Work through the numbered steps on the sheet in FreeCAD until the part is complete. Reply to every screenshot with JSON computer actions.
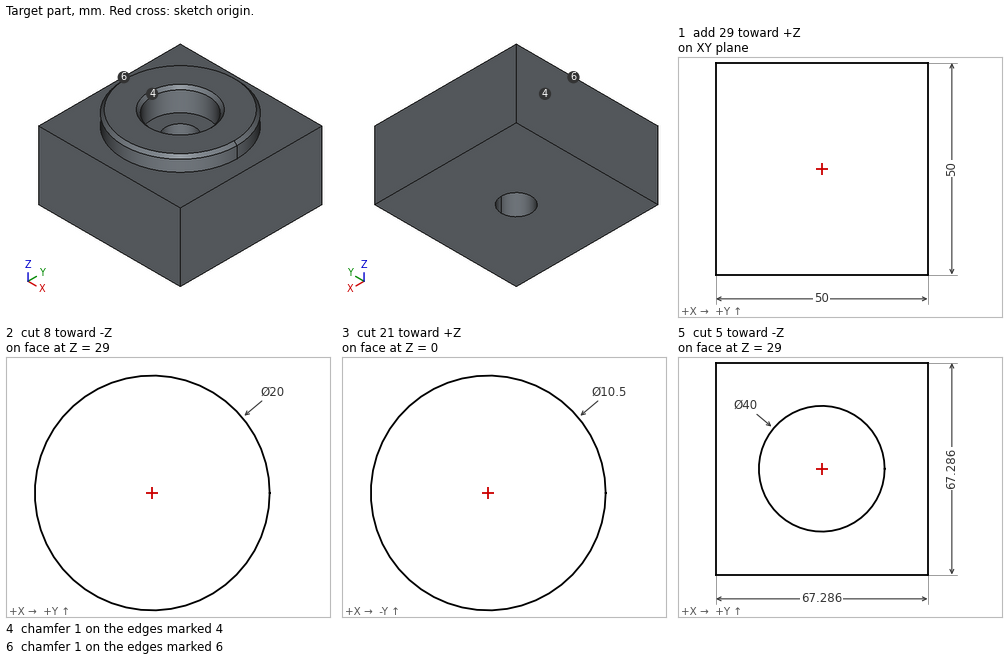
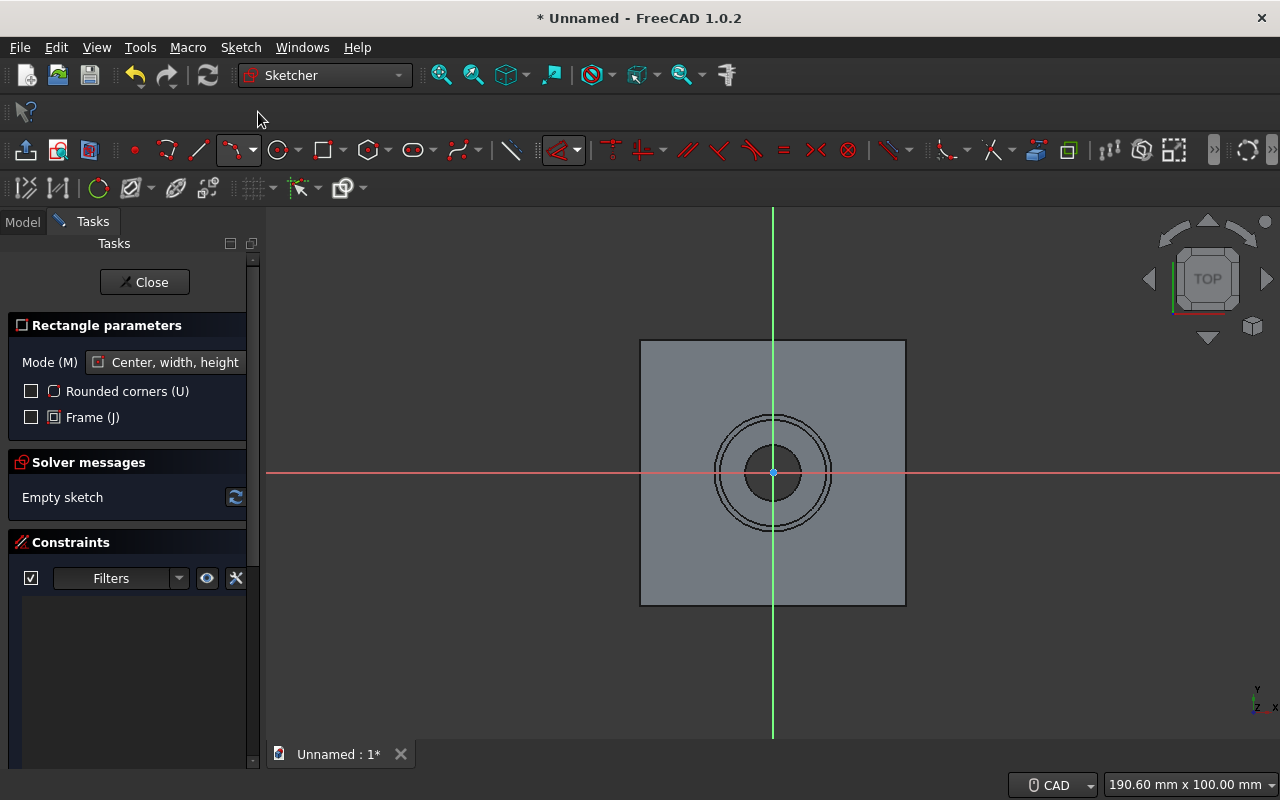
{"action": "left_click", "coordinate": [773, 473]}
{"action": "mouse_move", "coordinate": [952, 294]}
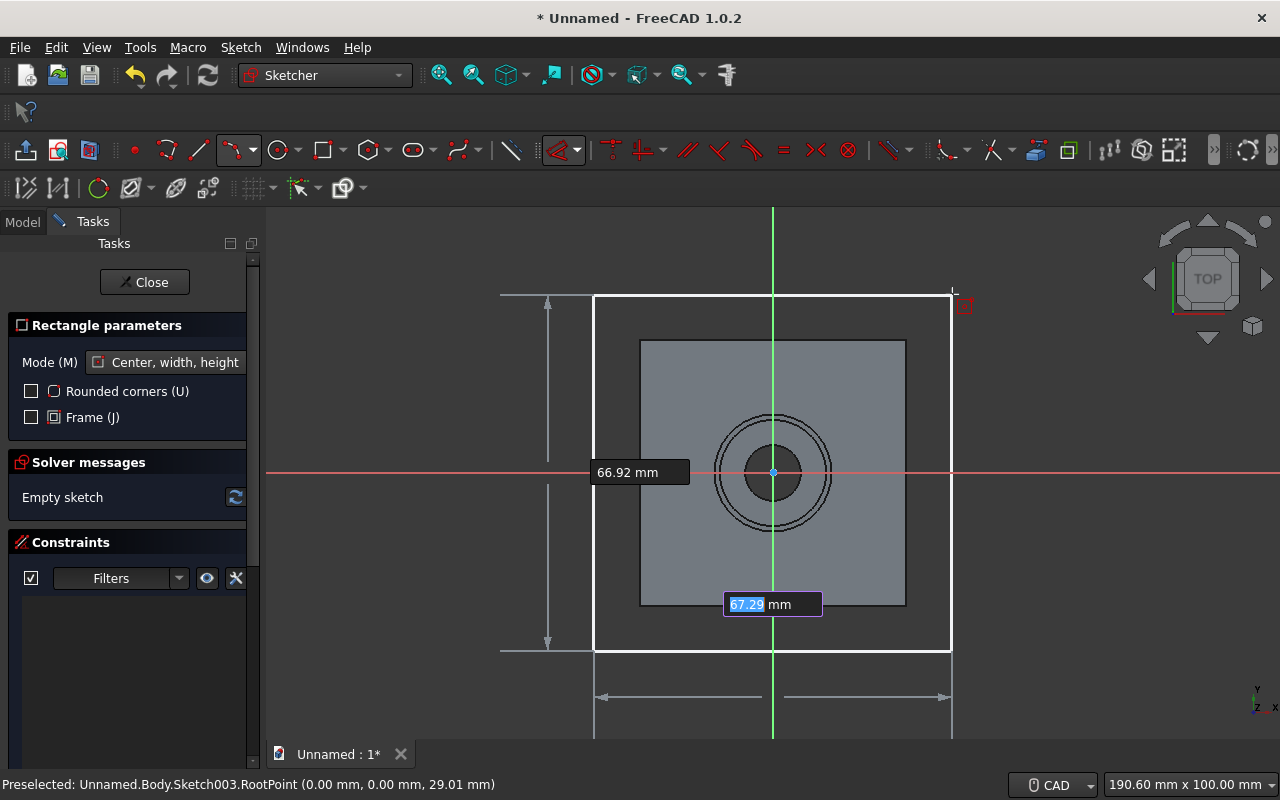
{"action": "type", "text": "67.286"}
{"action": "key", "text": "Tab"}
{"action": "type", "text": "67.286"}
{"action": "key", "text": "Return"}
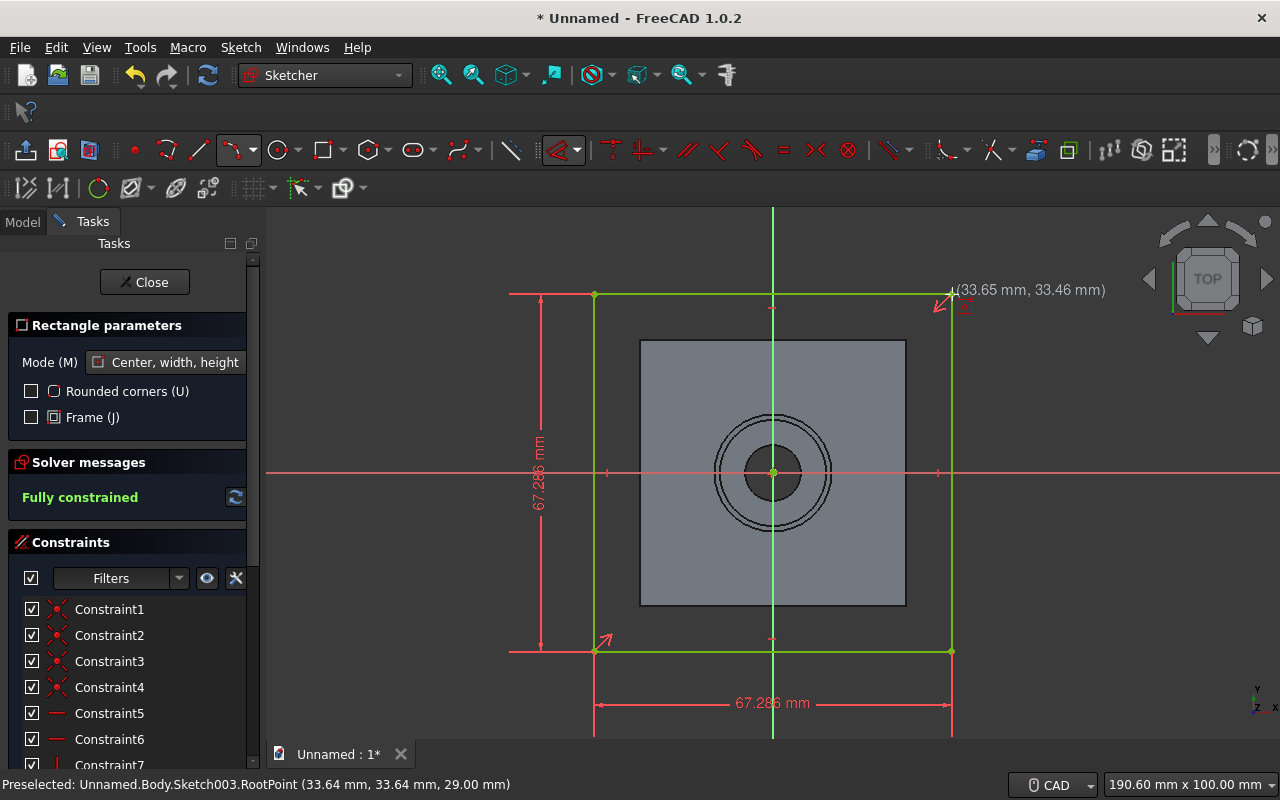
{"action": "left_click", "coordinate": [278, 150]}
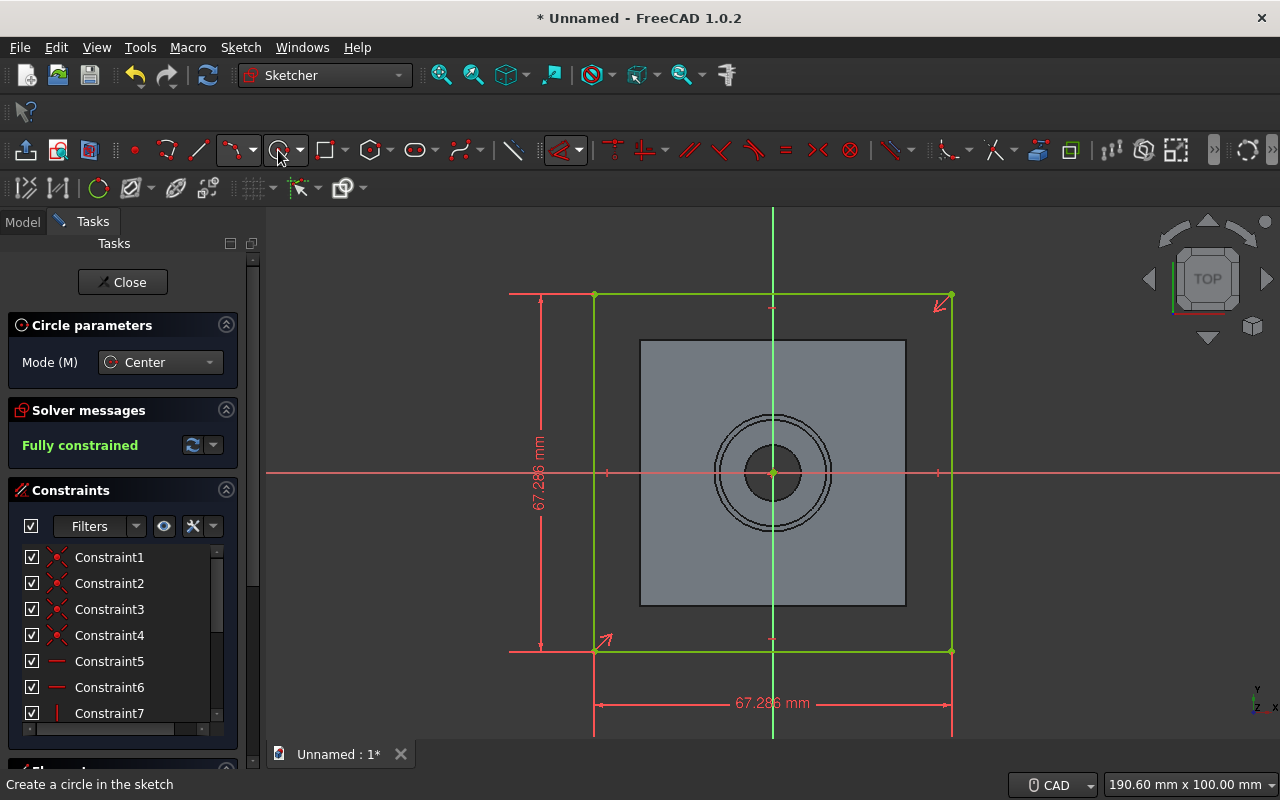
{"action": "left_click", "coordinate": [773, 473]}
{"action": "mouse_move", "coordinate": [848, 398]}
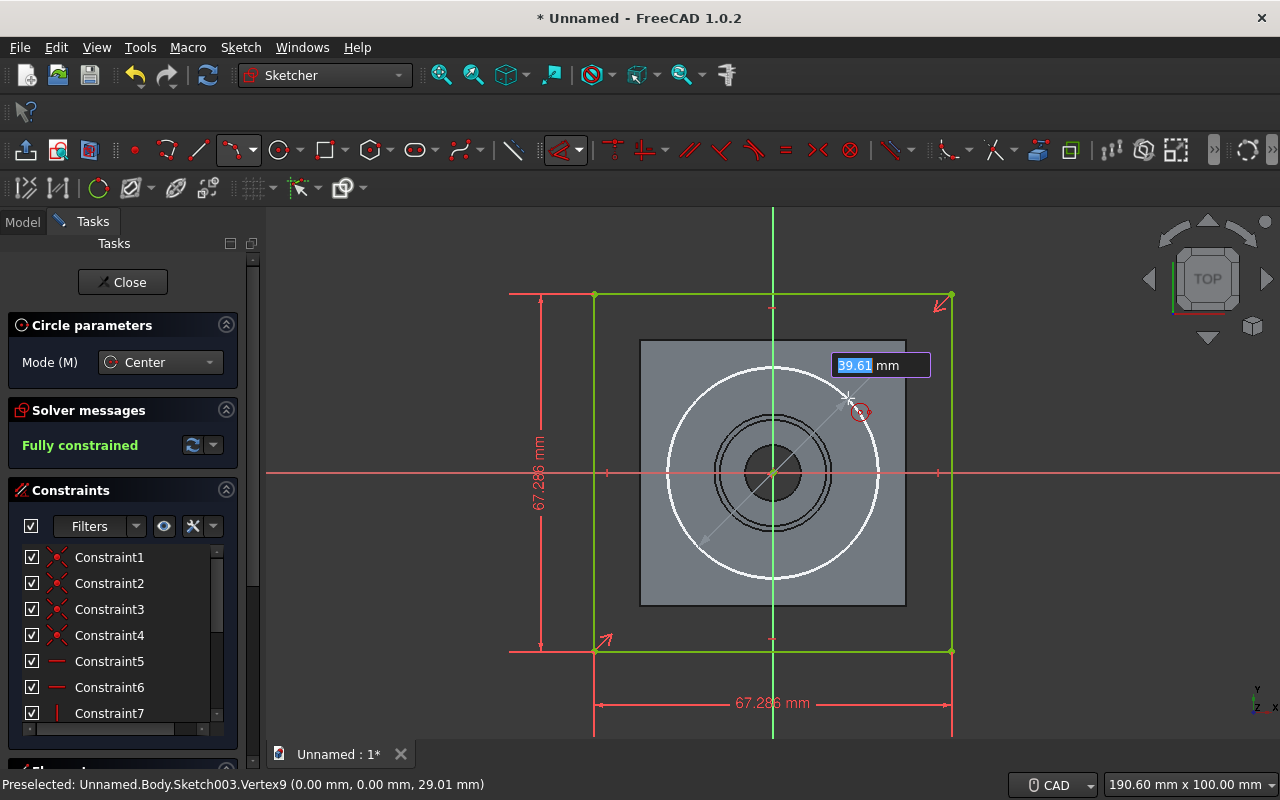
{"action": "type", "text": "40"}
{"action": "key", "text": "Return"}
{"action": "key", "text": "Escape"}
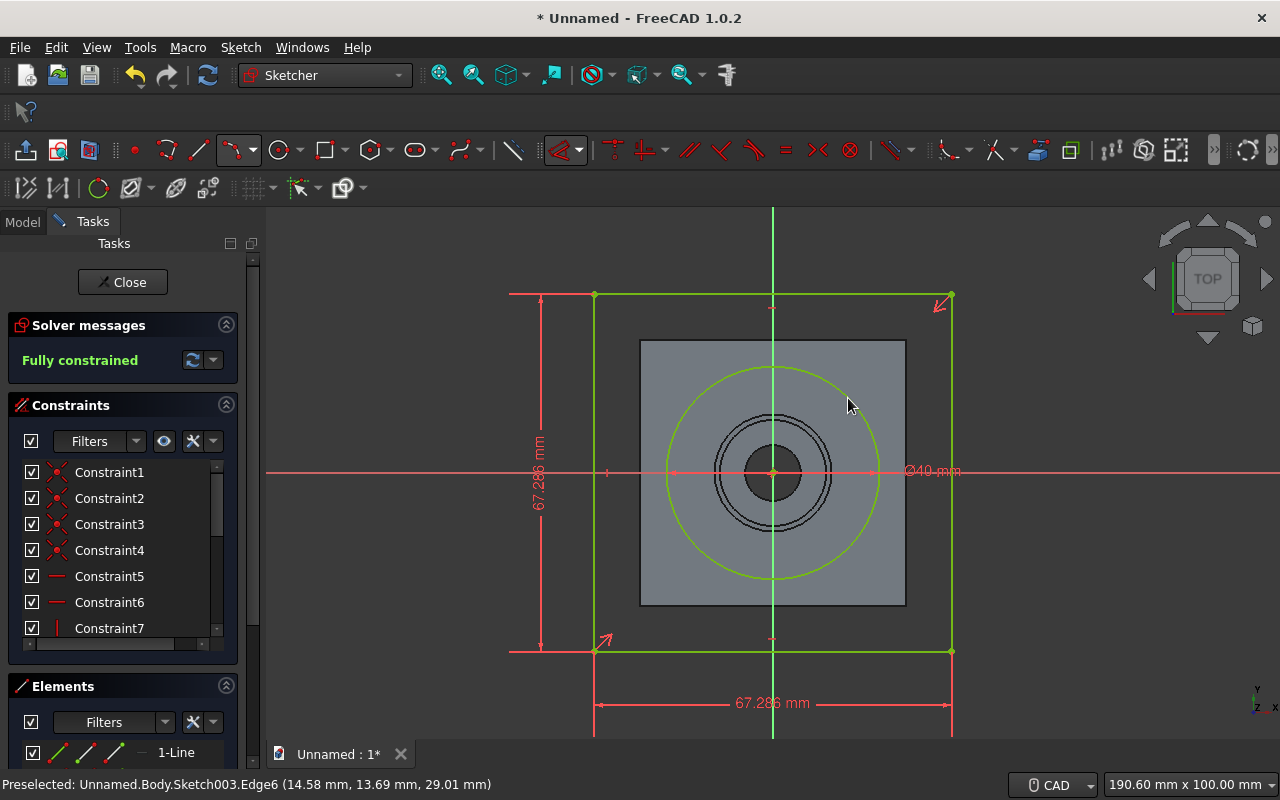
{"action": "left_click", "coordinate": [123, 282]}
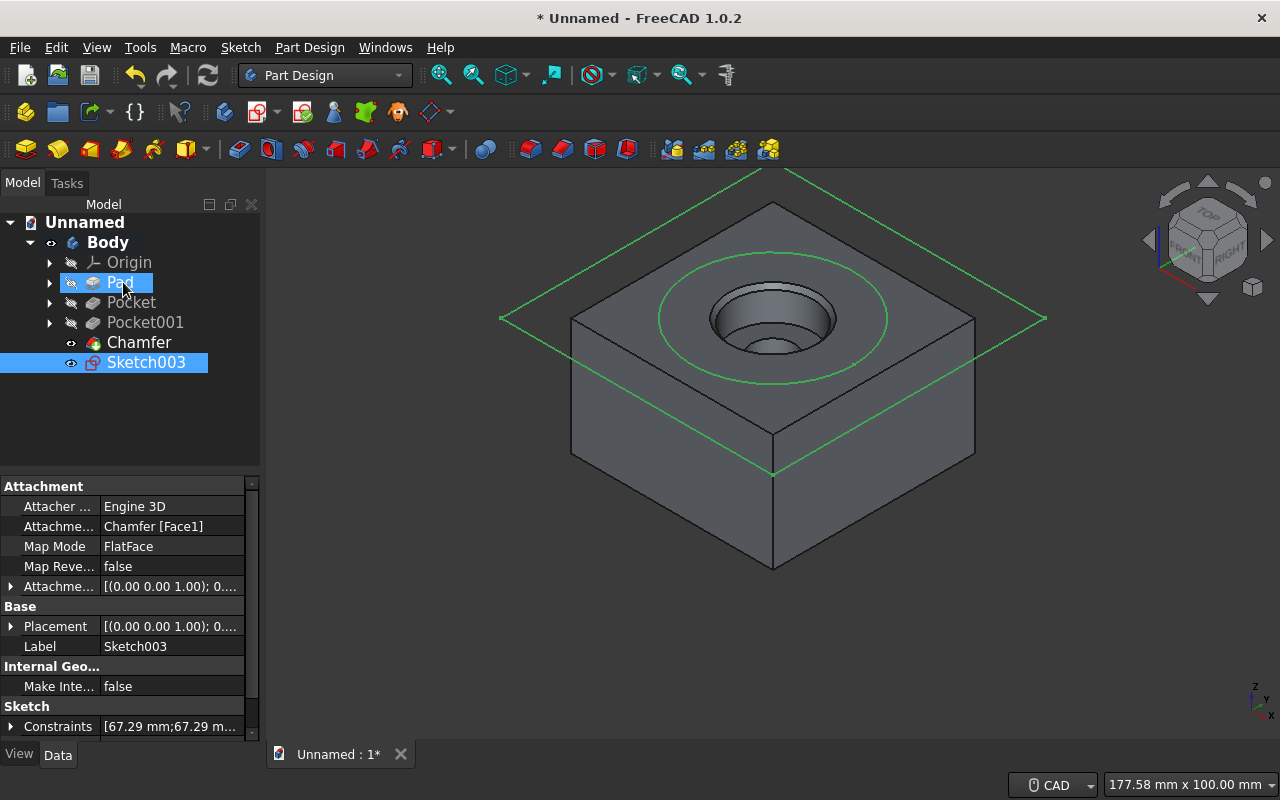
{"action": "left_click", "coordinate": [240, 150]}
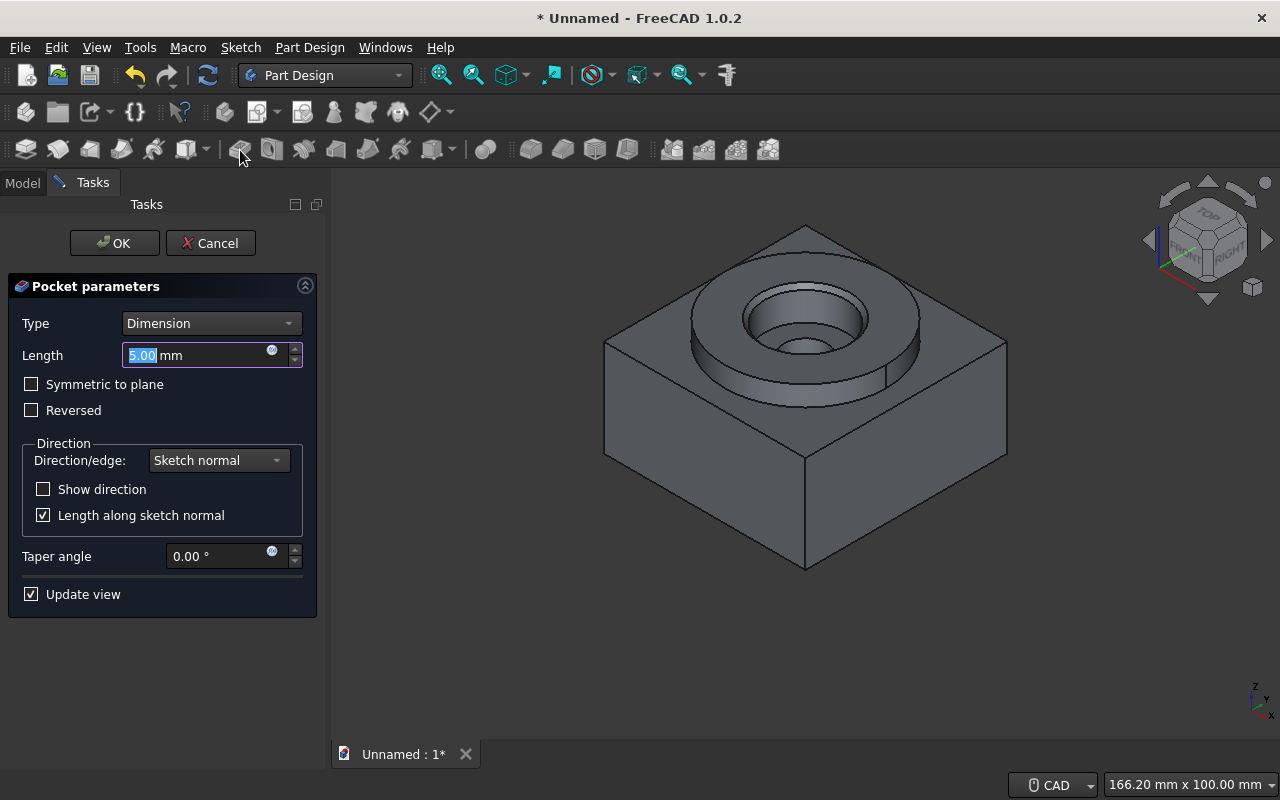
{"action": "type", "text": "5"}
{"action": "key", "text": "Tab"}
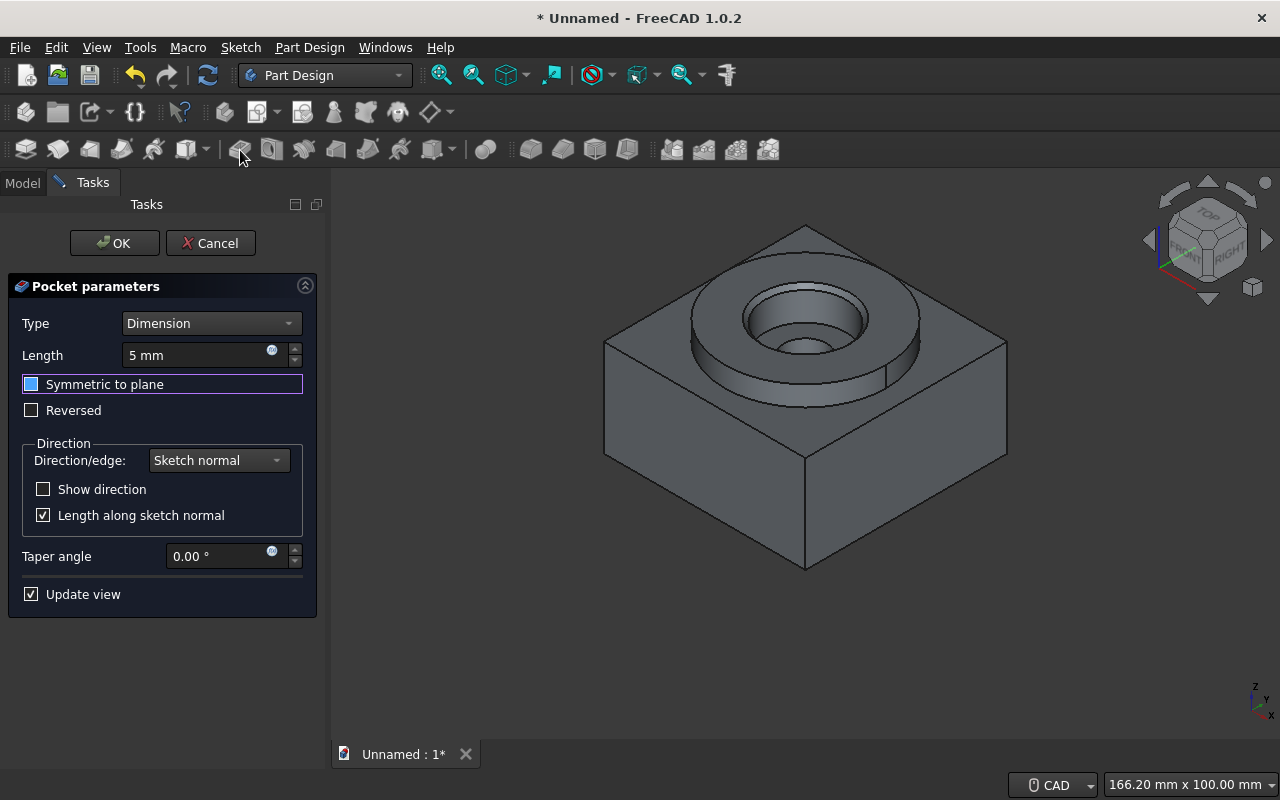
{"action": "left_click", "coordinate": [115, 243]}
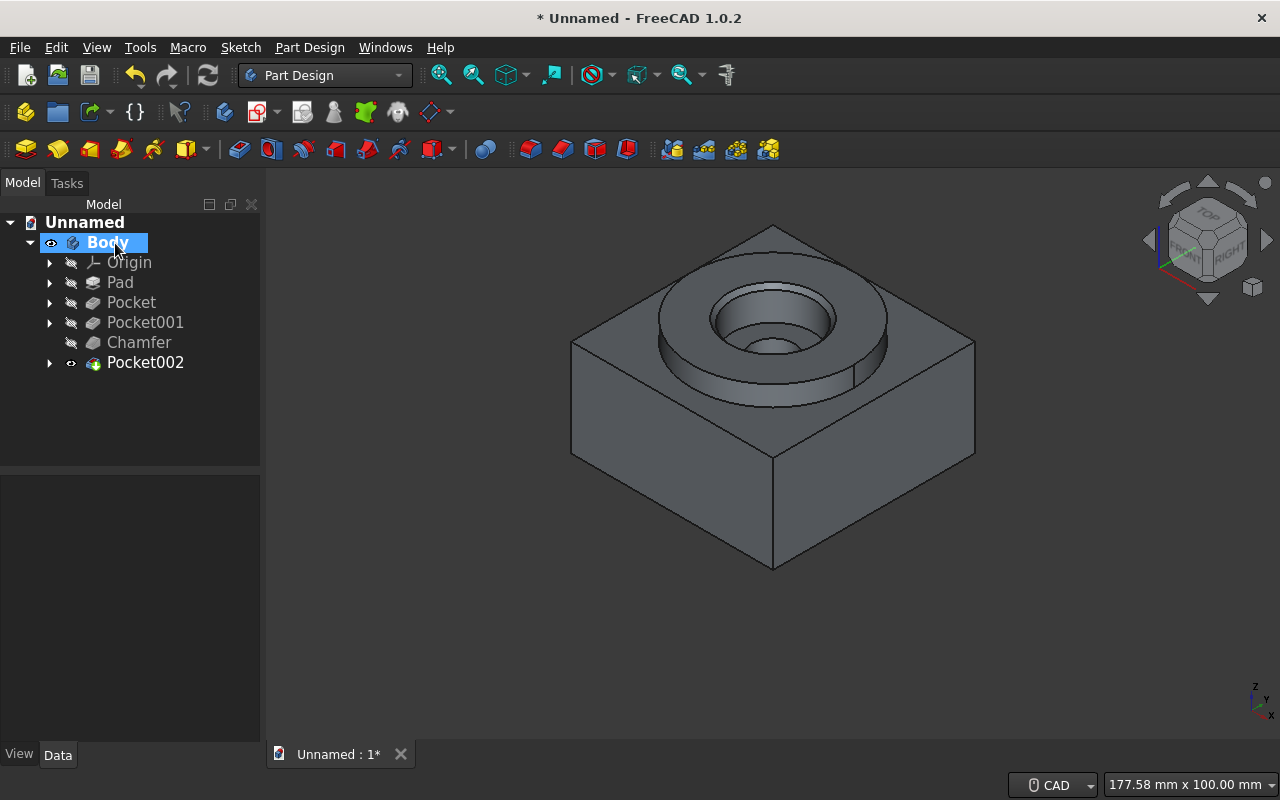
{"action": "left_click", "coordinate": [660, 307]}